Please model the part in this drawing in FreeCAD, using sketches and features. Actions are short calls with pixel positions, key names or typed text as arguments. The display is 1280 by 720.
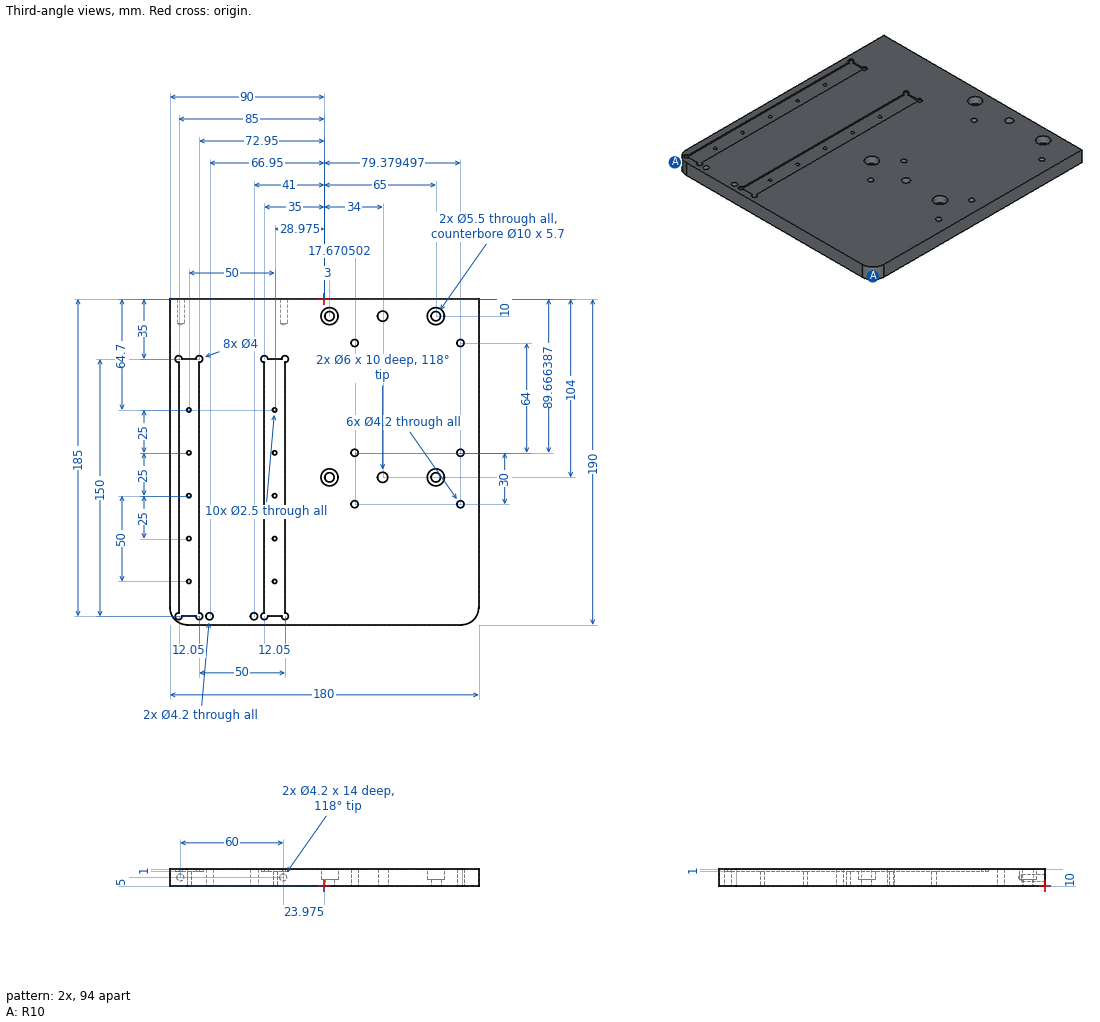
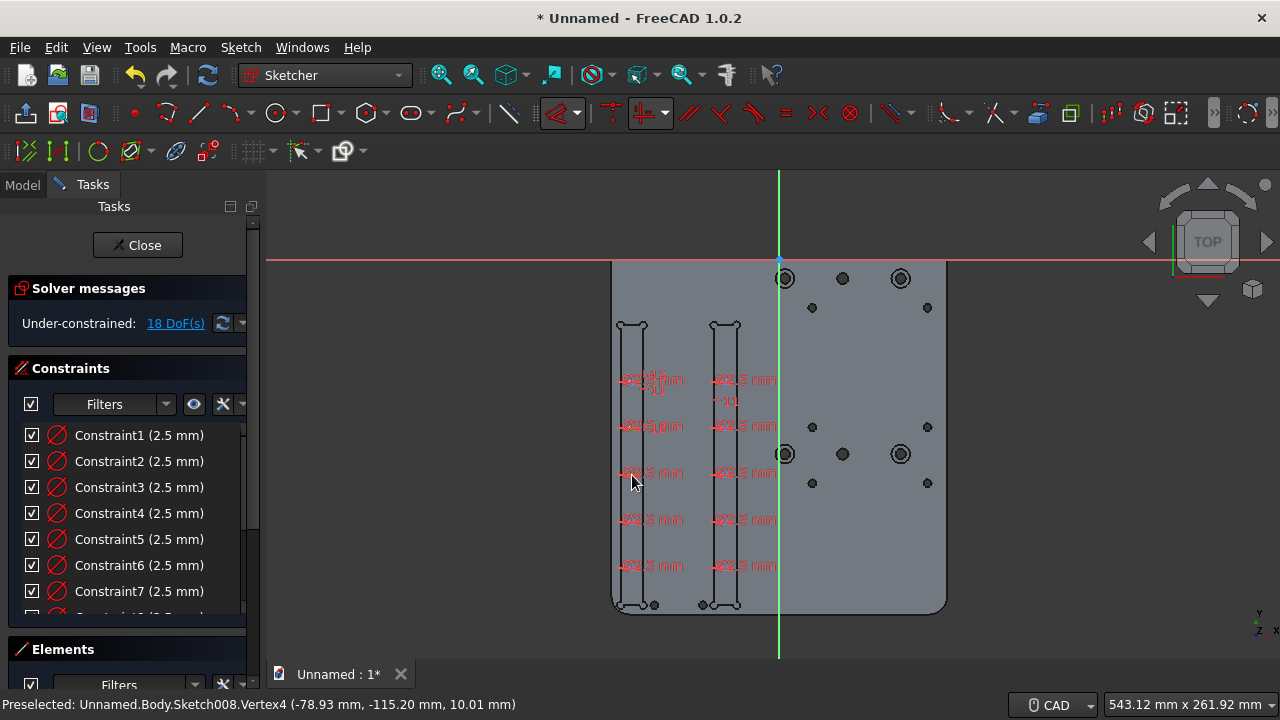
key(v)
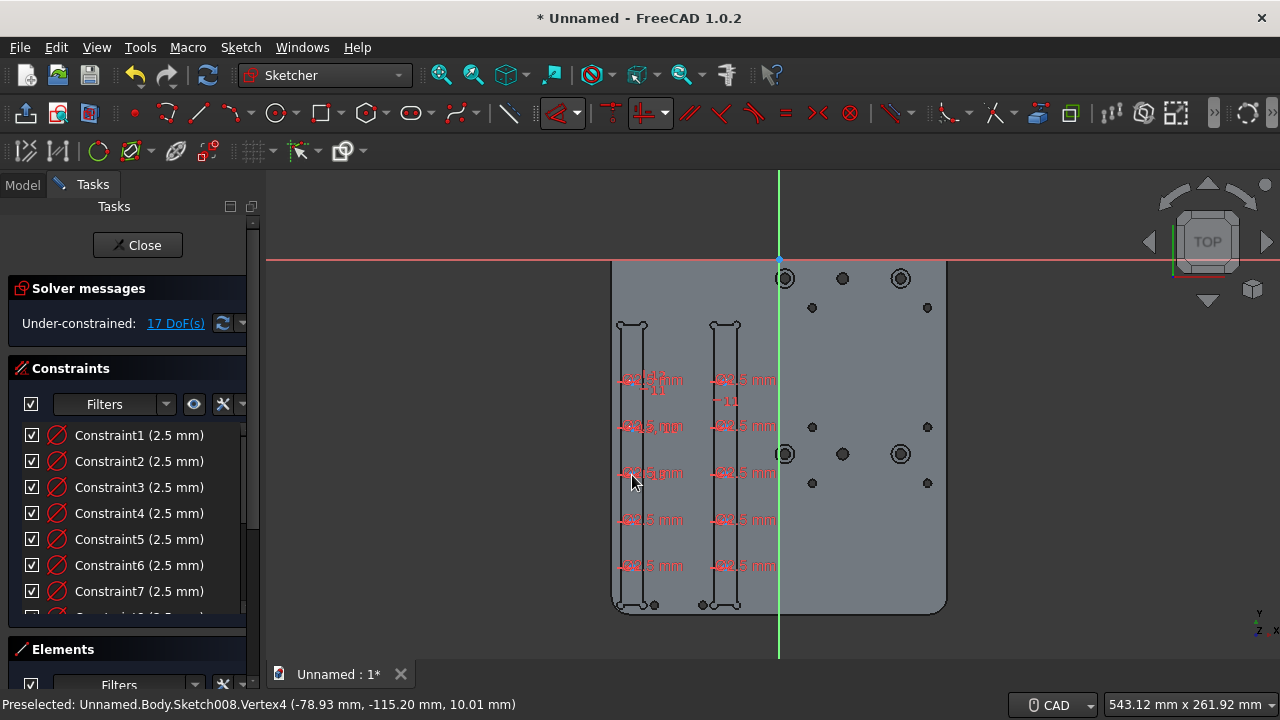
click(632, 475)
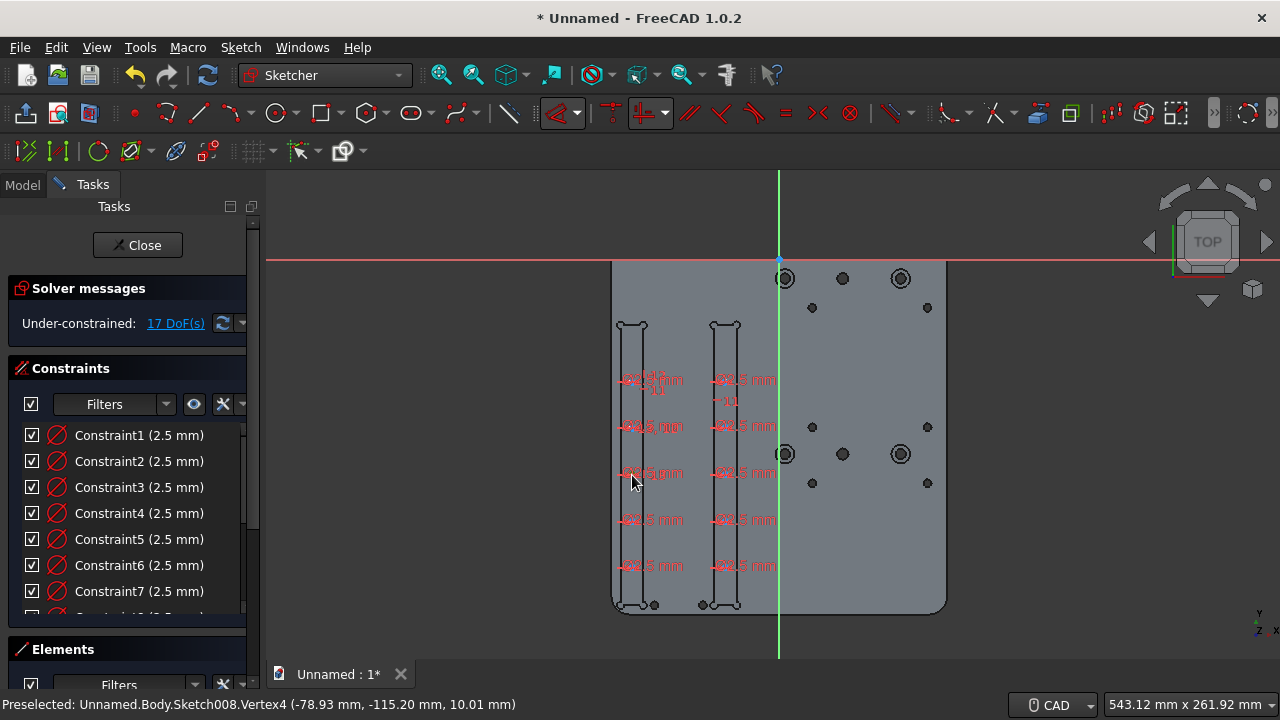
click(632, 568)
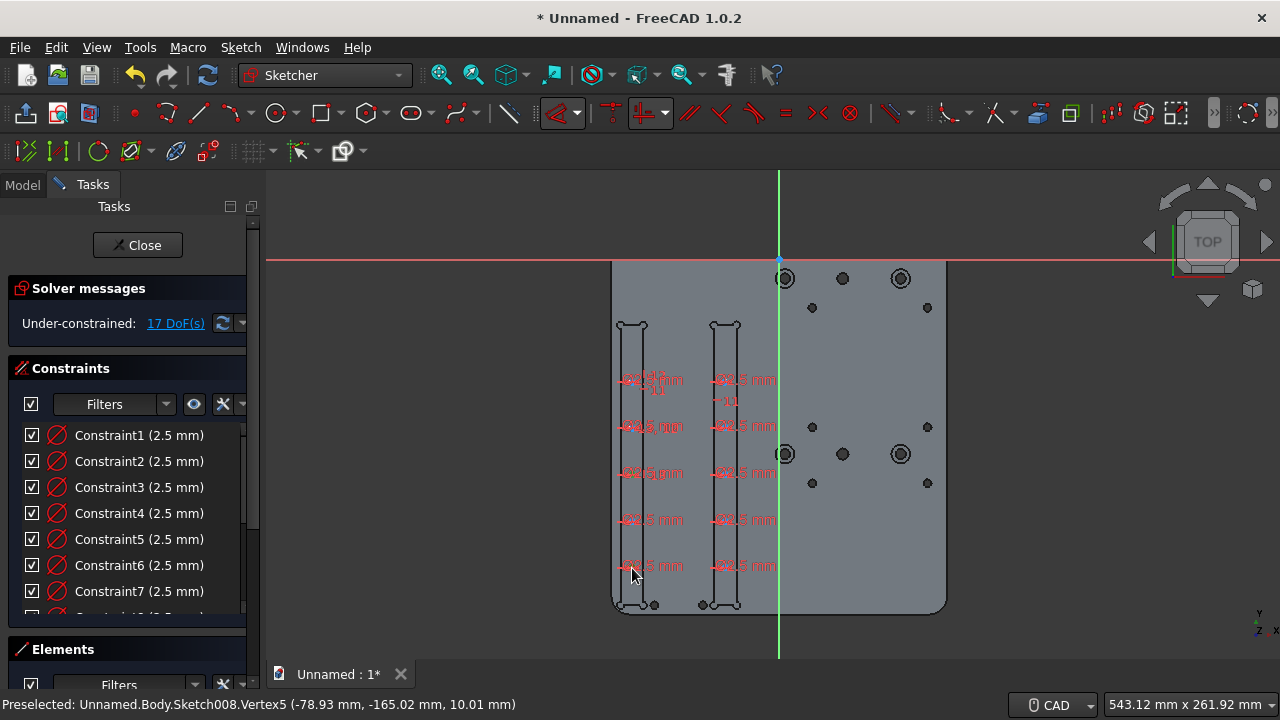
key(v)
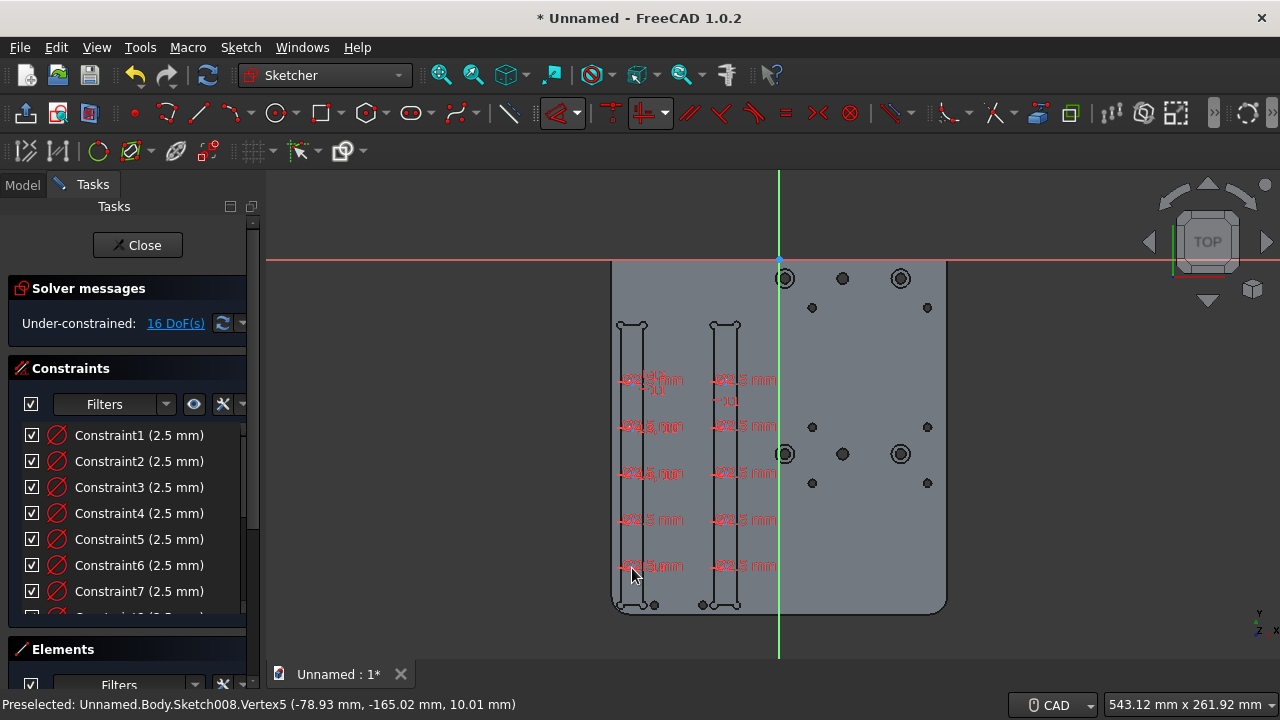
click(632, 475)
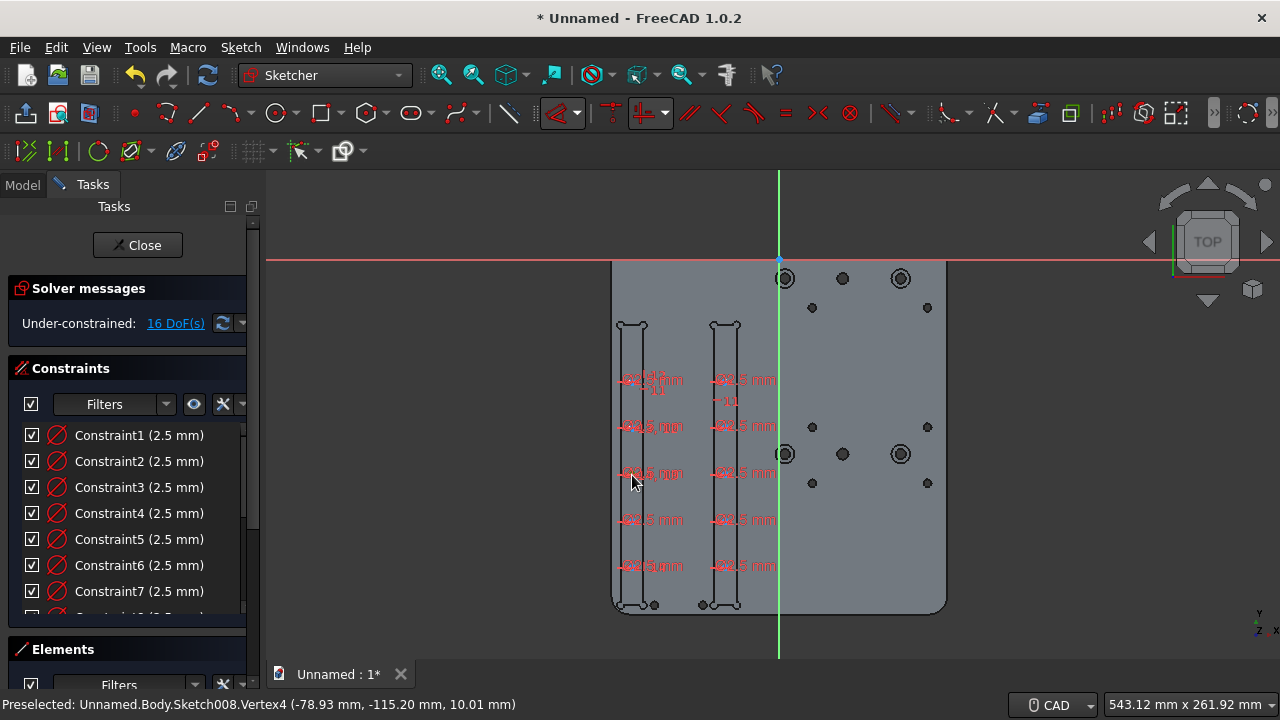
click(632, 522)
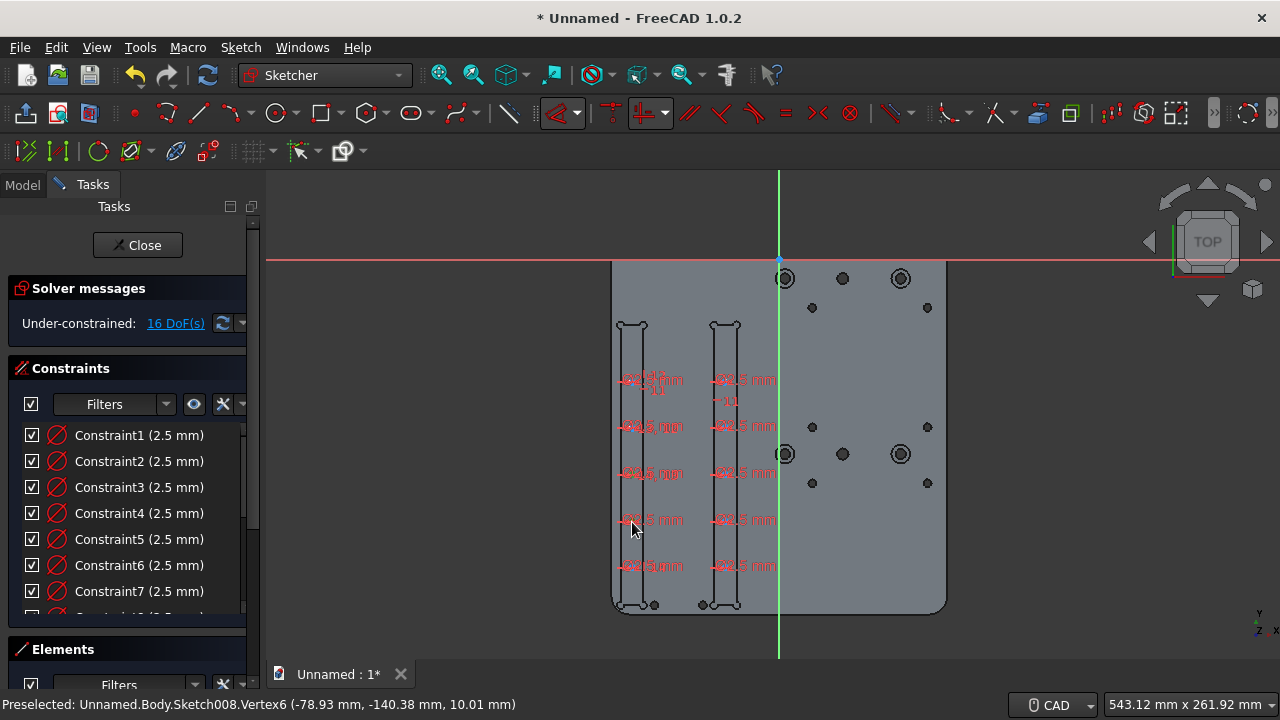
key(v)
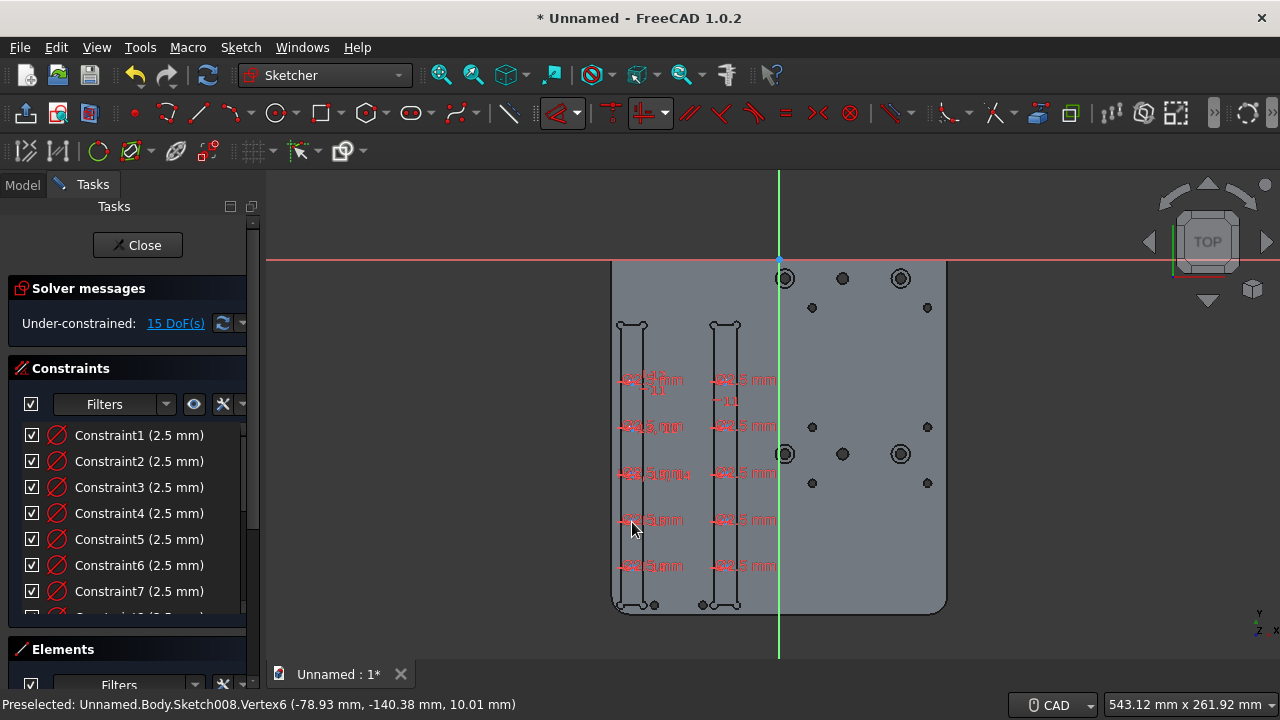
click(725, 382)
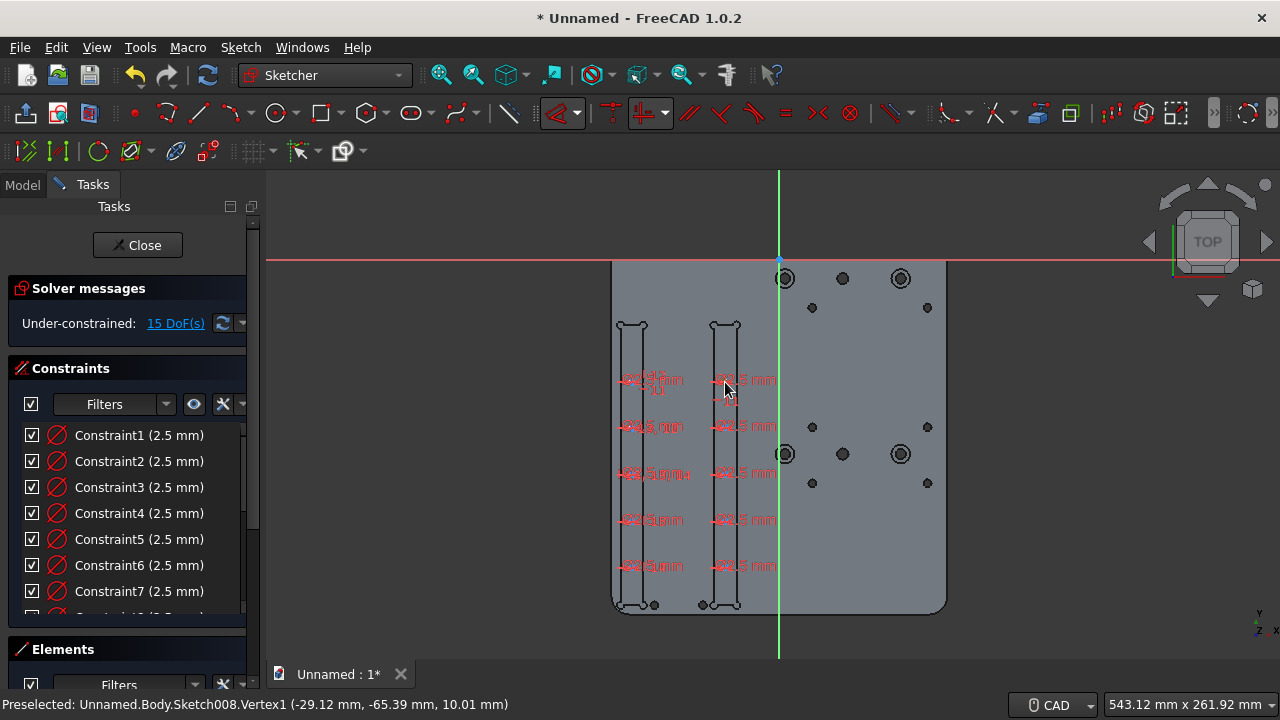
click(725, 568)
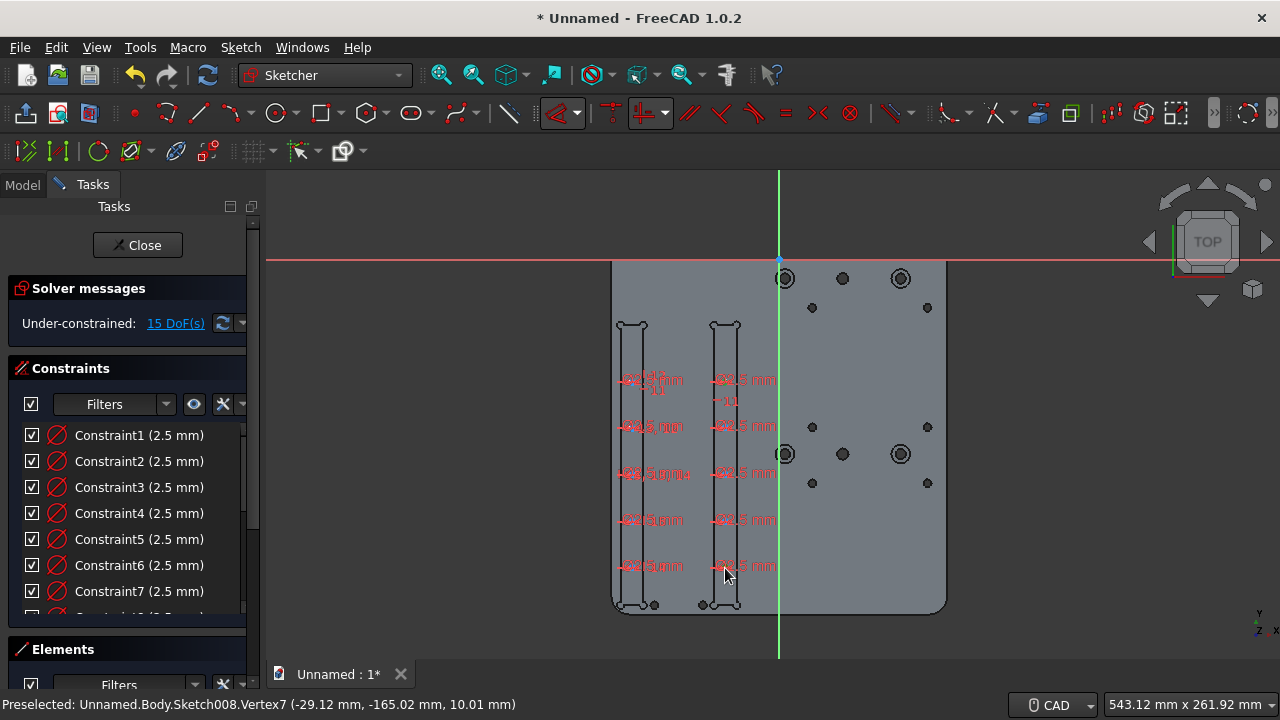
key(v)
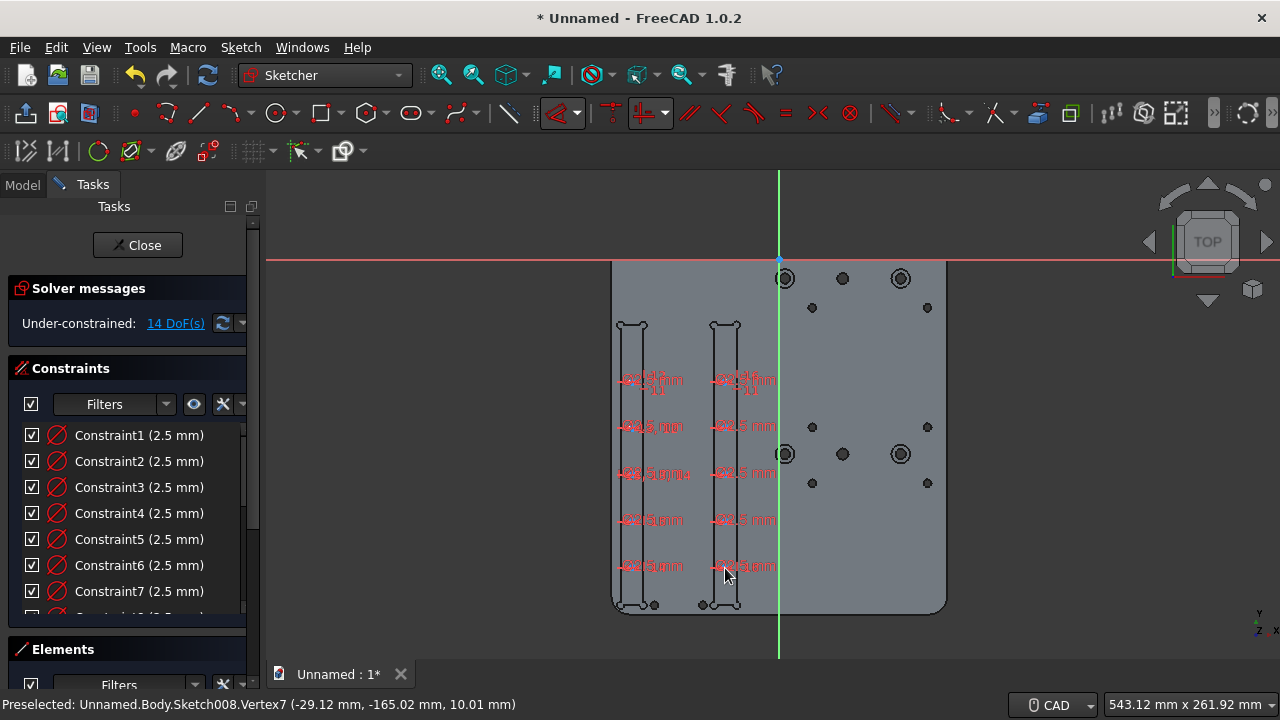
click(632, 568)